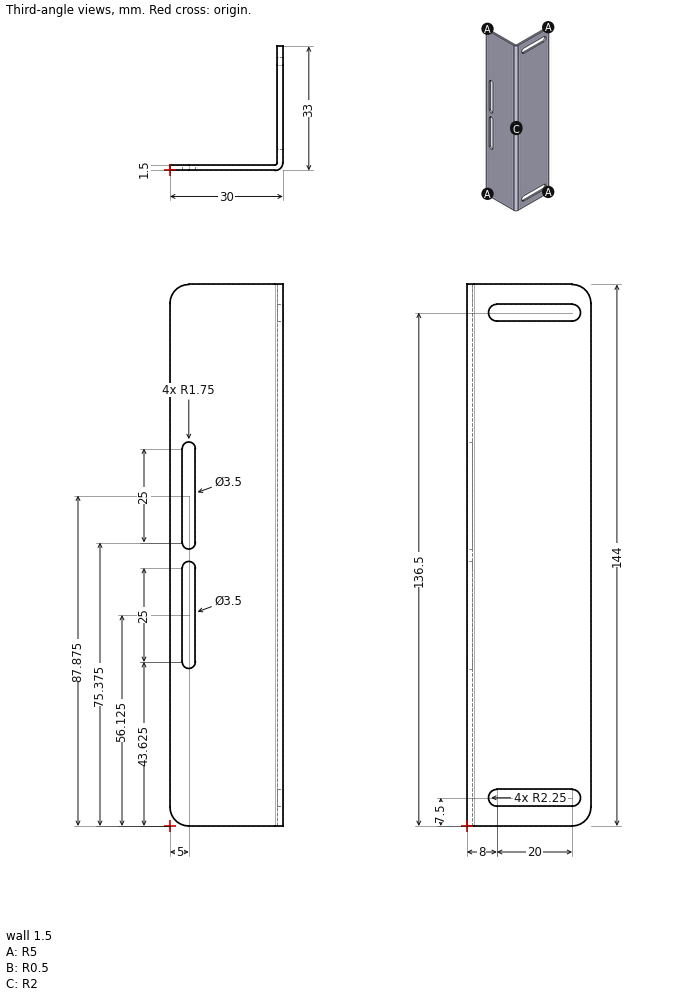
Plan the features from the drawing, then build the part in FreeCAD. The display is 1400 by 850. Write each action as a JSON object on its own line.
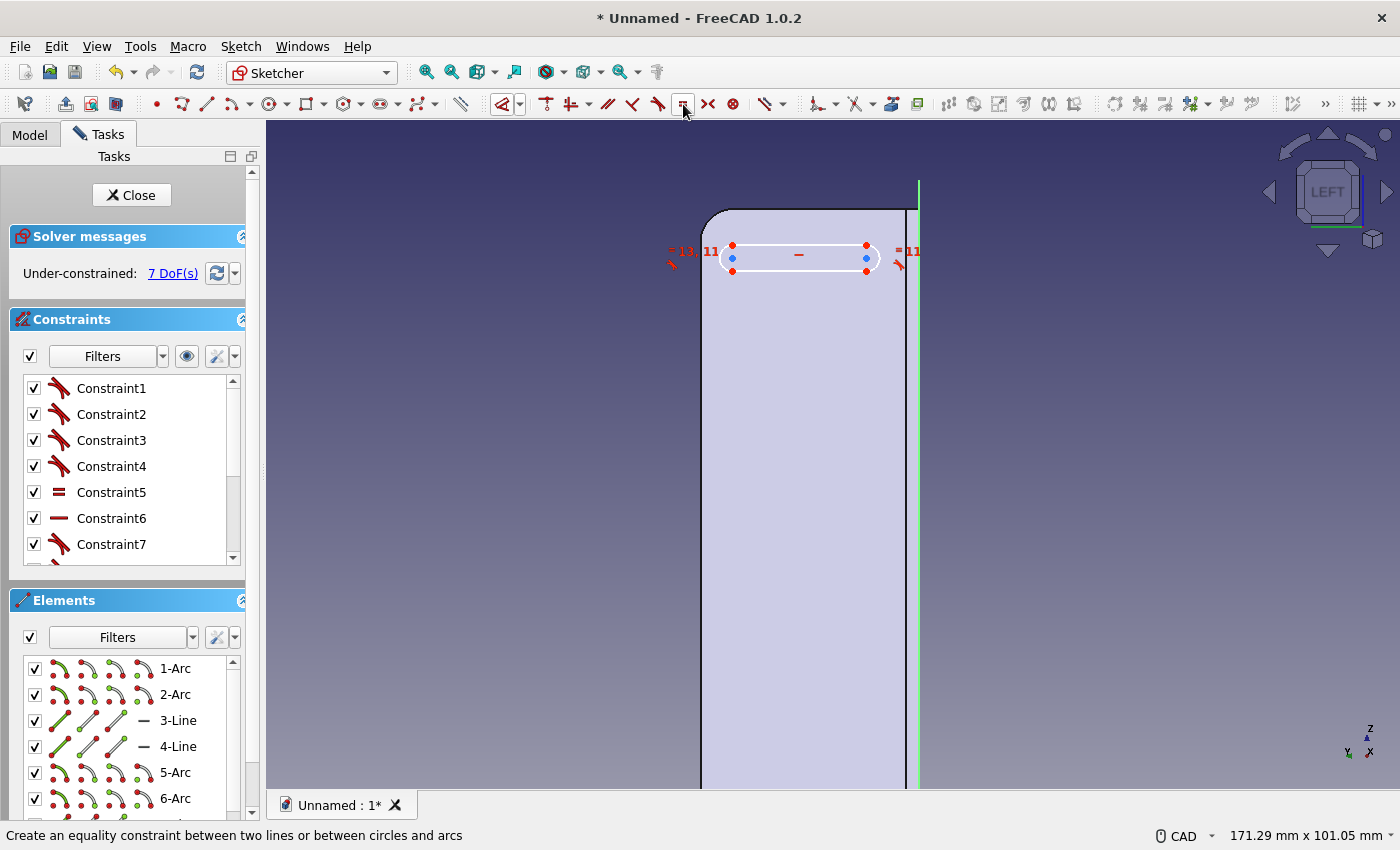
{"action": "scroll", "coordinate": [720, 252], "scroll_direction": "down", "scroll_amount": 4}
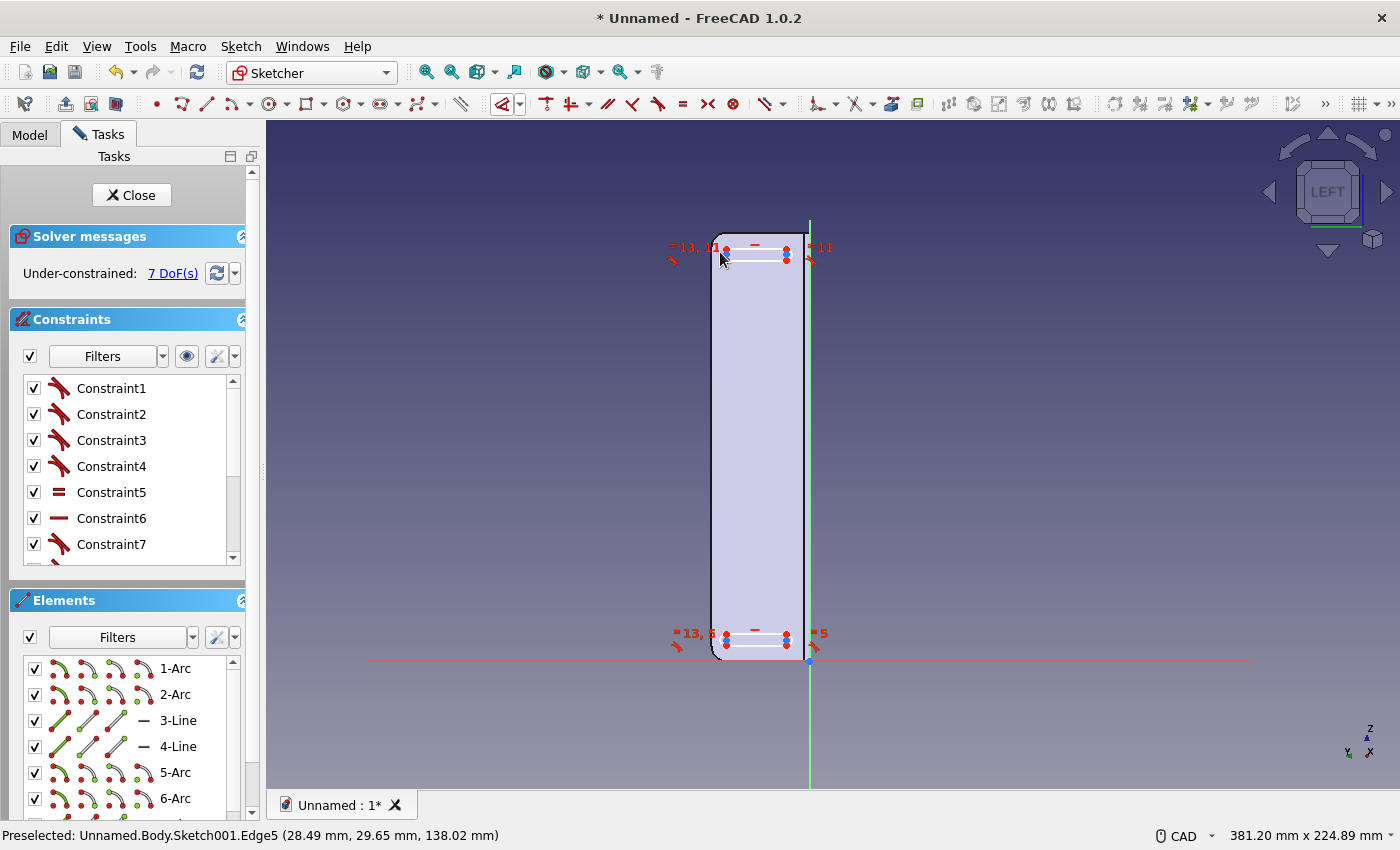
{"action": "scroll", "coordinate": [721, 637], "scroll_direction": "up", "scroll_amount": 9}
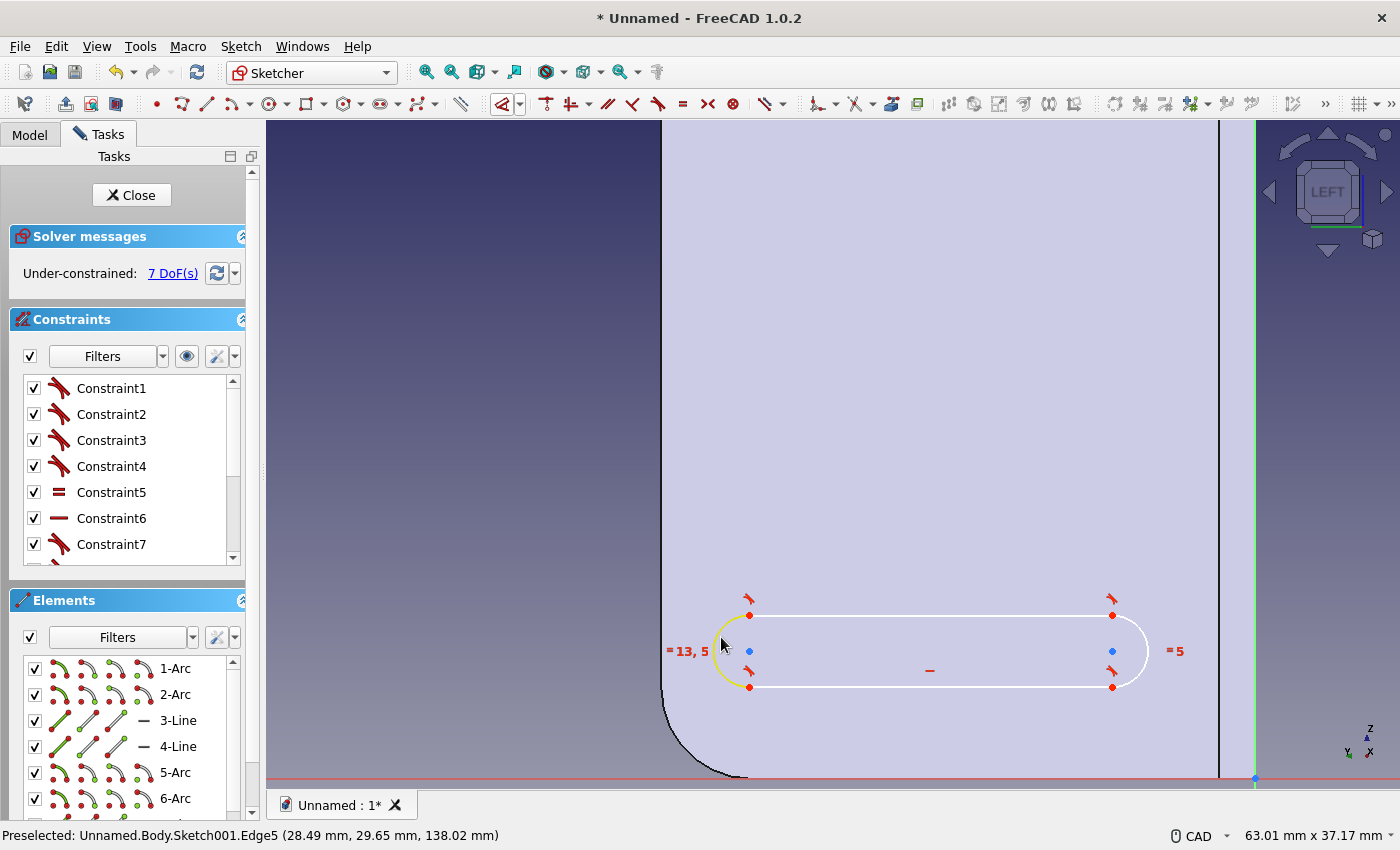
{"action": "left_click", "coordinate": [720, 630]}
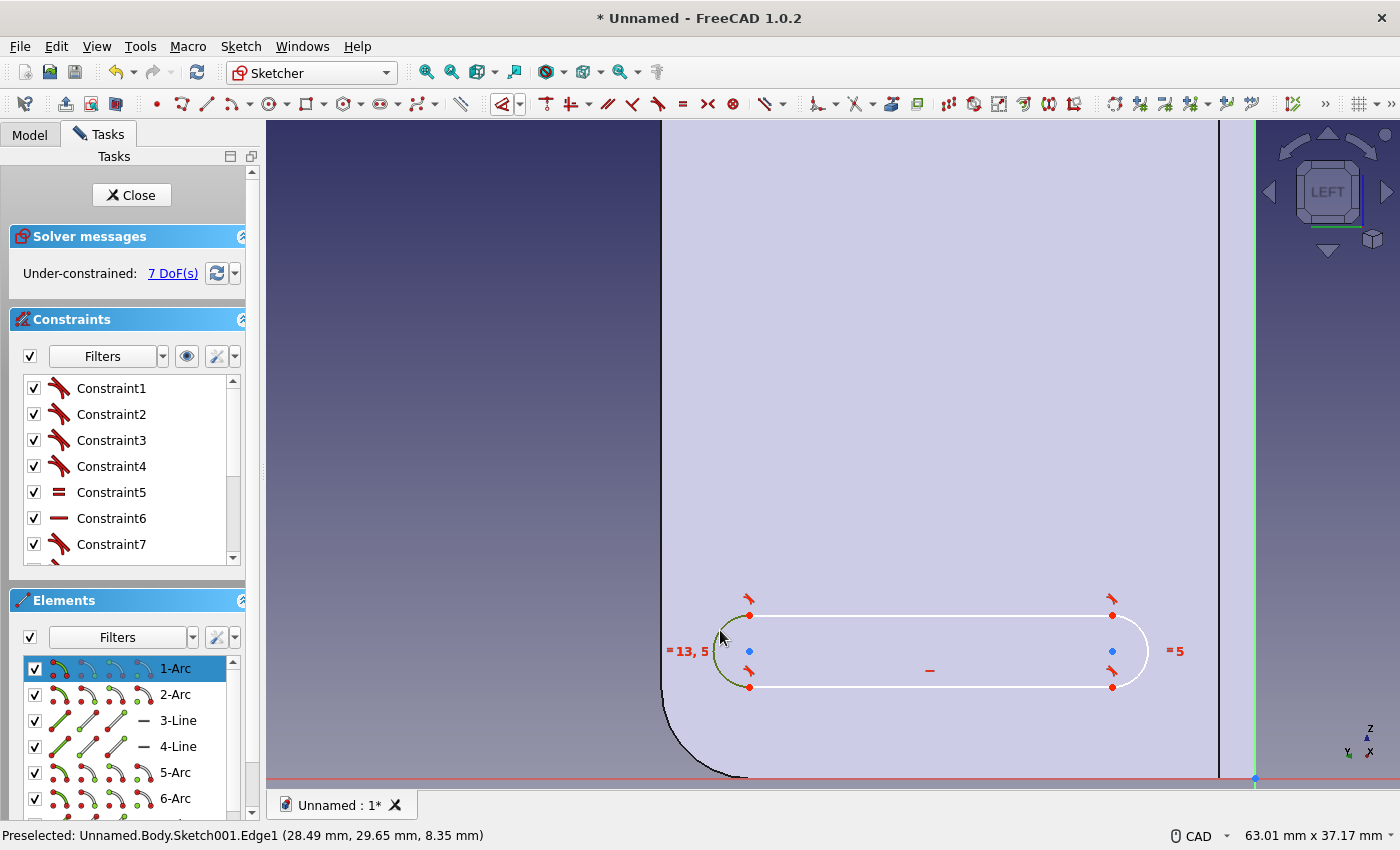
{"action": "key", "text": "k r"}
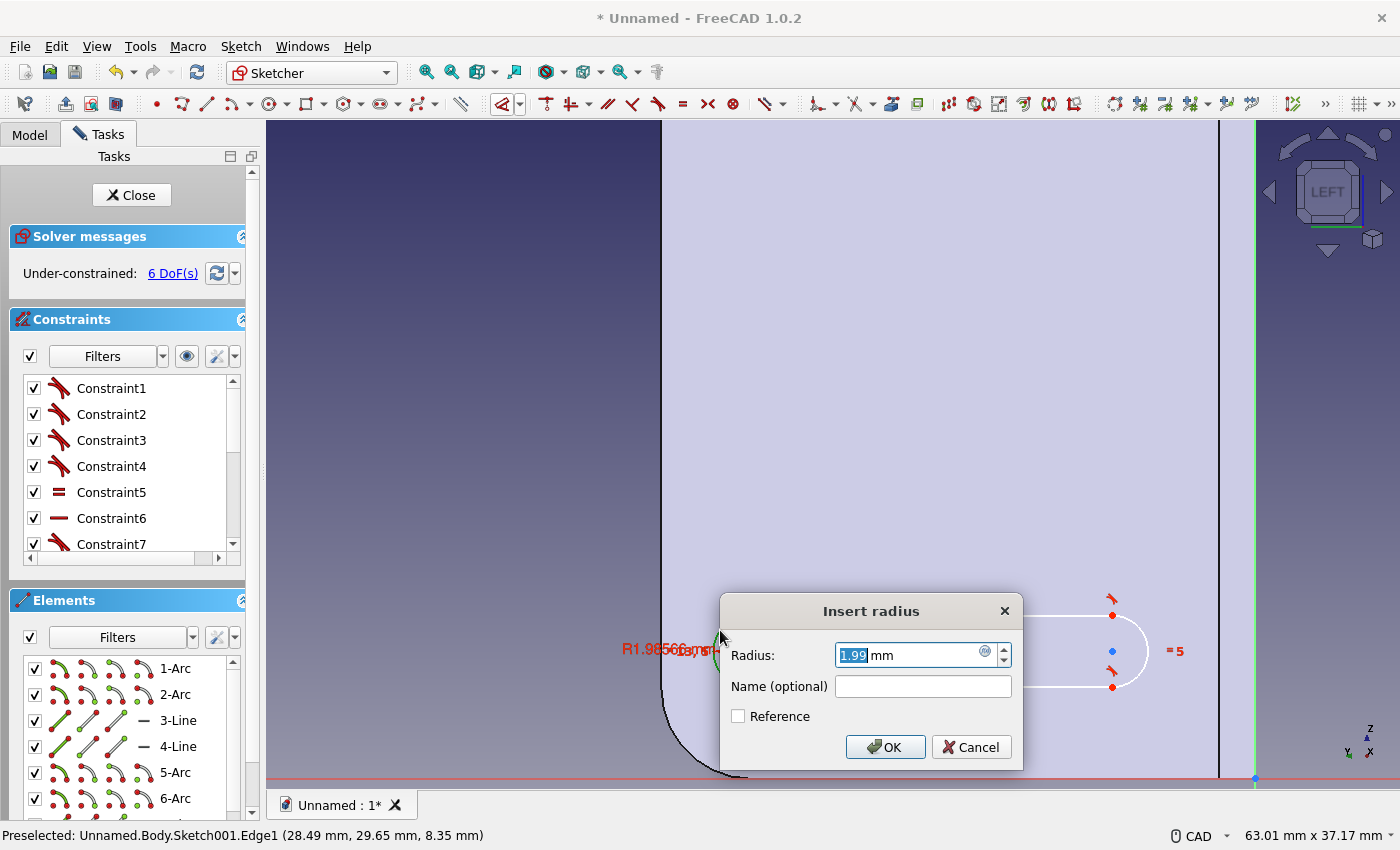
{"action": "type", "text": "2.25"}
{"action": "key", "text": "Return"}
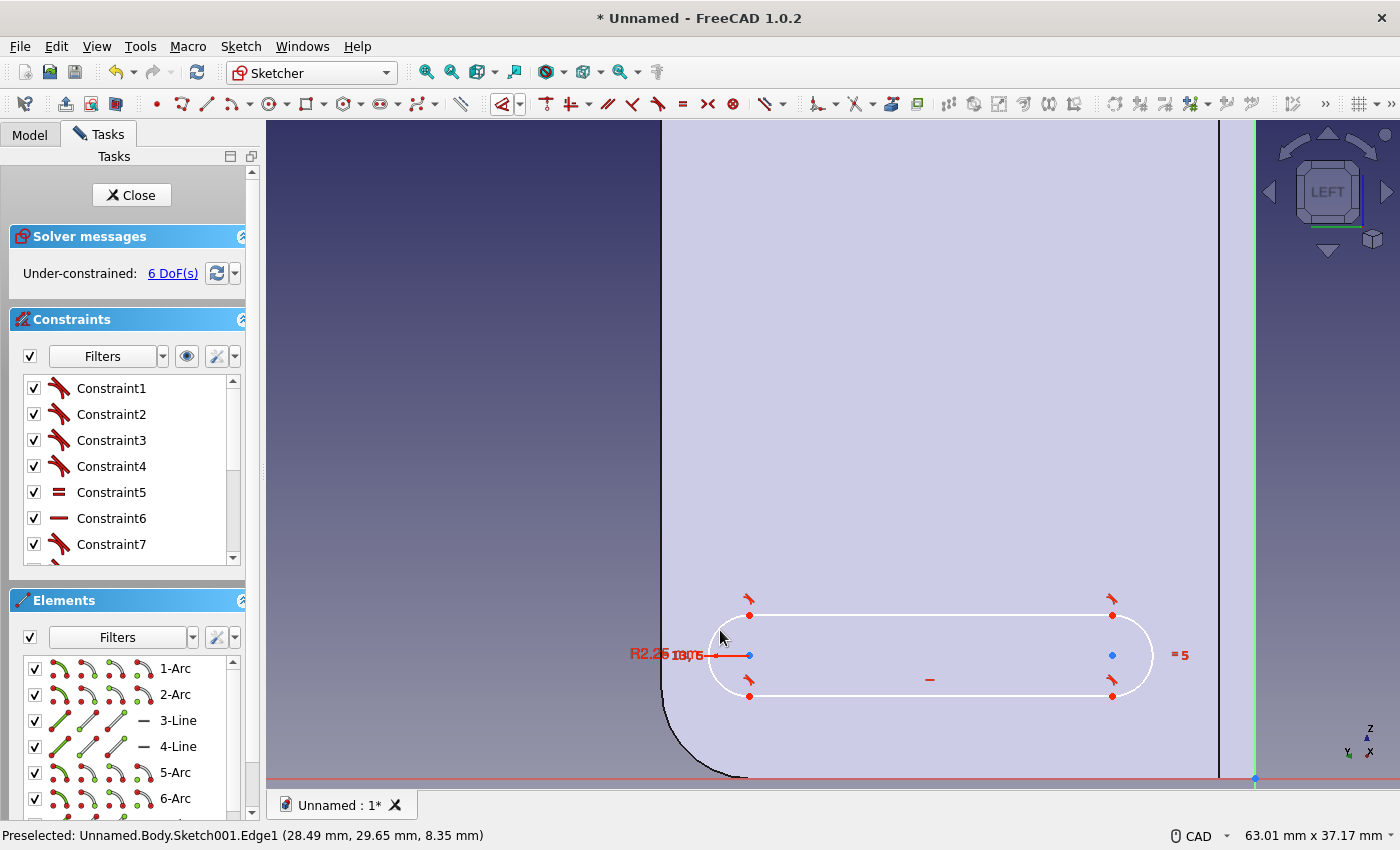
{"action": "scroll", "coordinate": [721, 638], "scroll_direction": "down", "scroll_amount": 9}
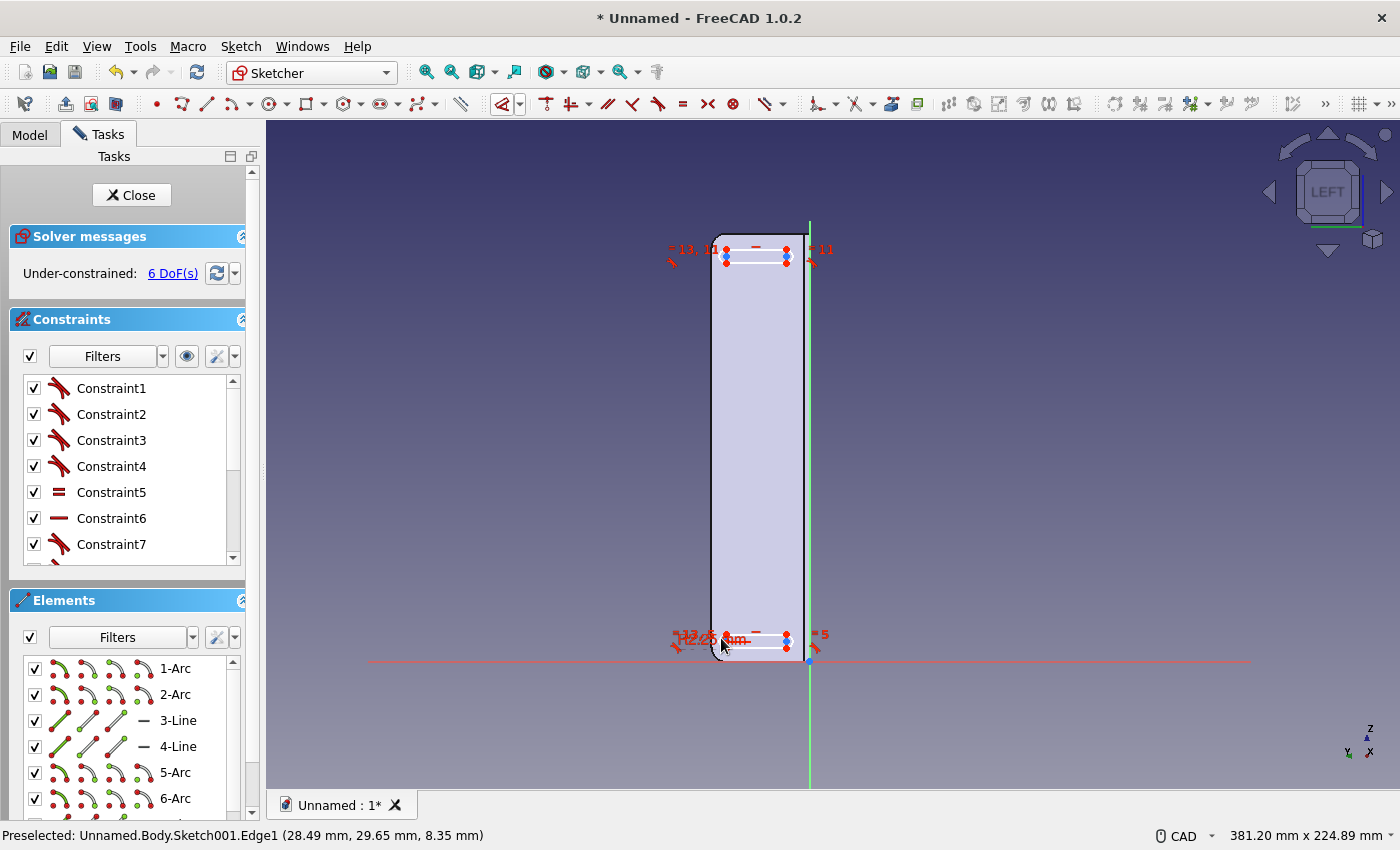
{"action": "left_click", "coordinate": [744, 635]}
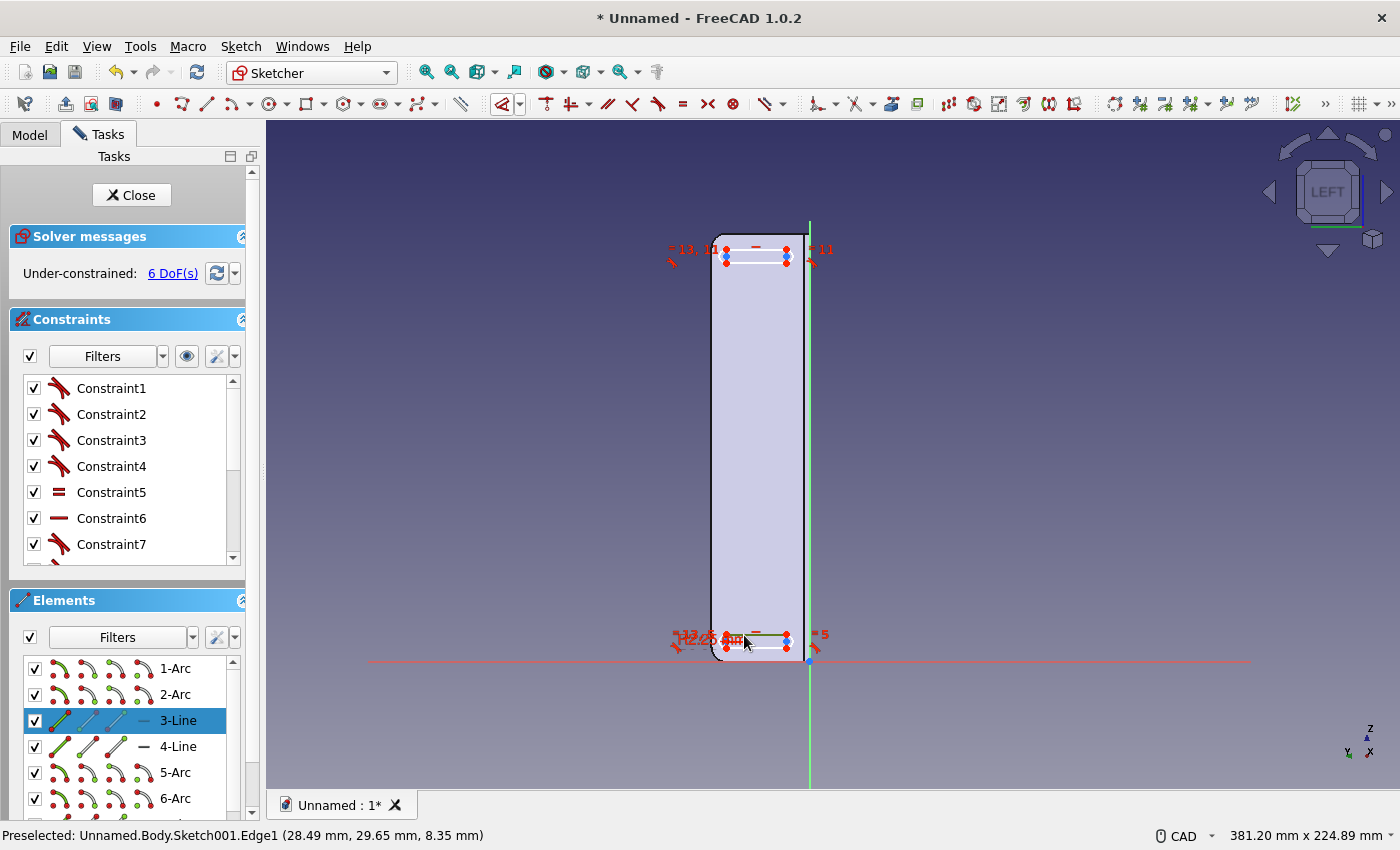
{"action": "left_click", "coordinate": [520, 104]}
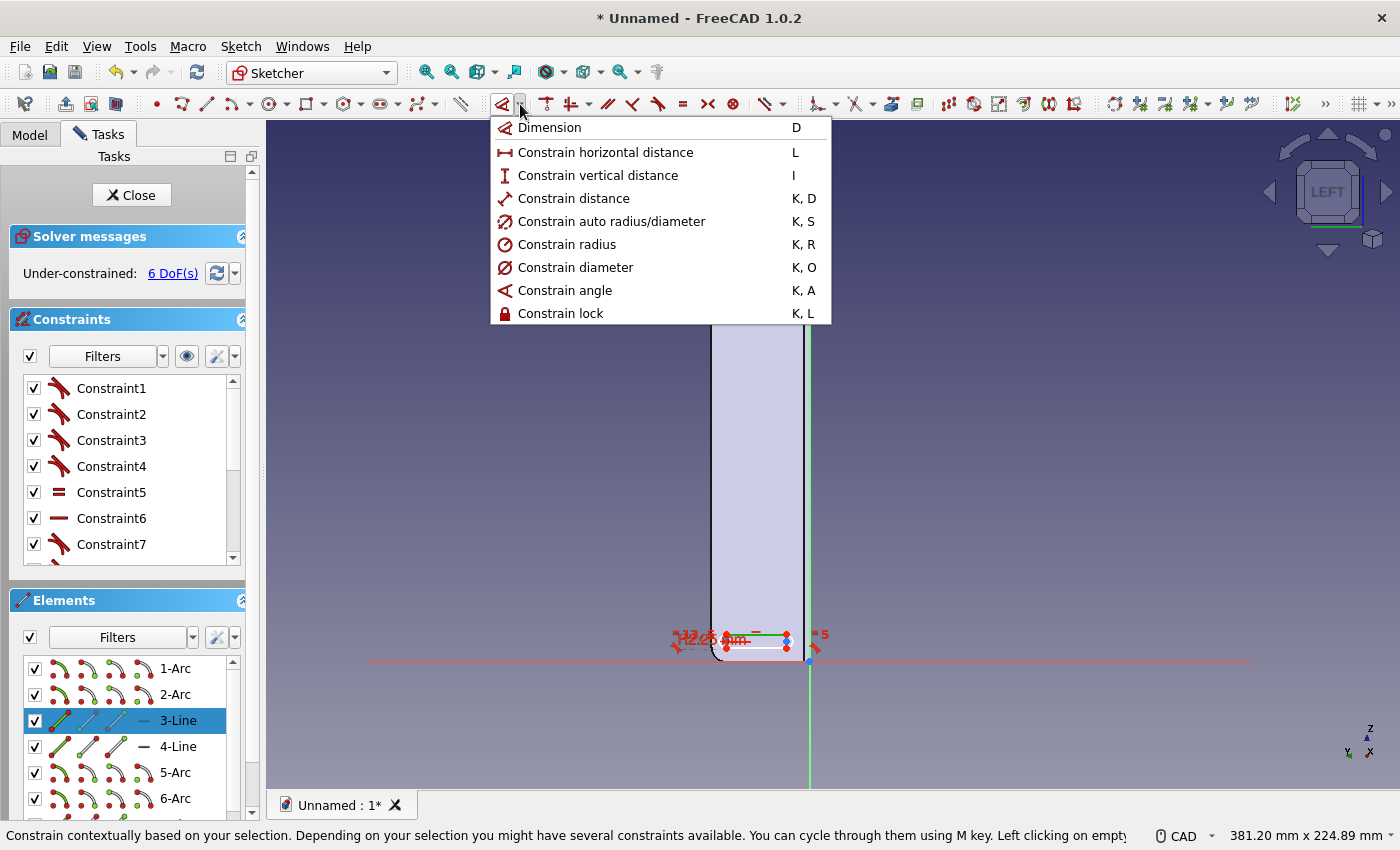
{"action": "left_click", "coordinate": [661, 152]}